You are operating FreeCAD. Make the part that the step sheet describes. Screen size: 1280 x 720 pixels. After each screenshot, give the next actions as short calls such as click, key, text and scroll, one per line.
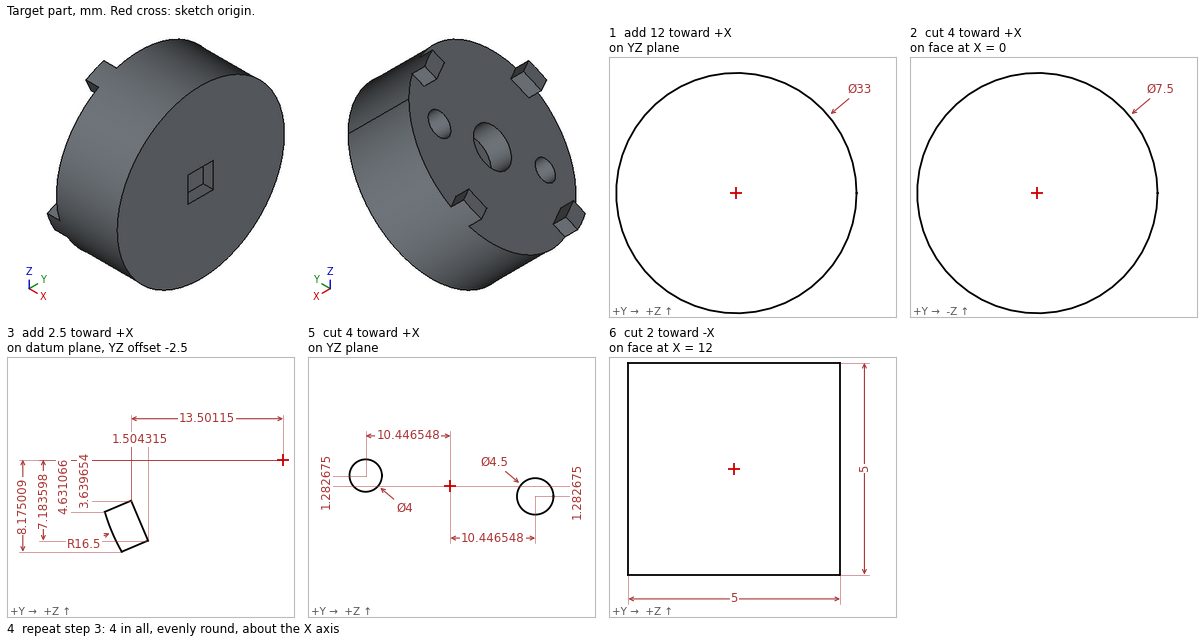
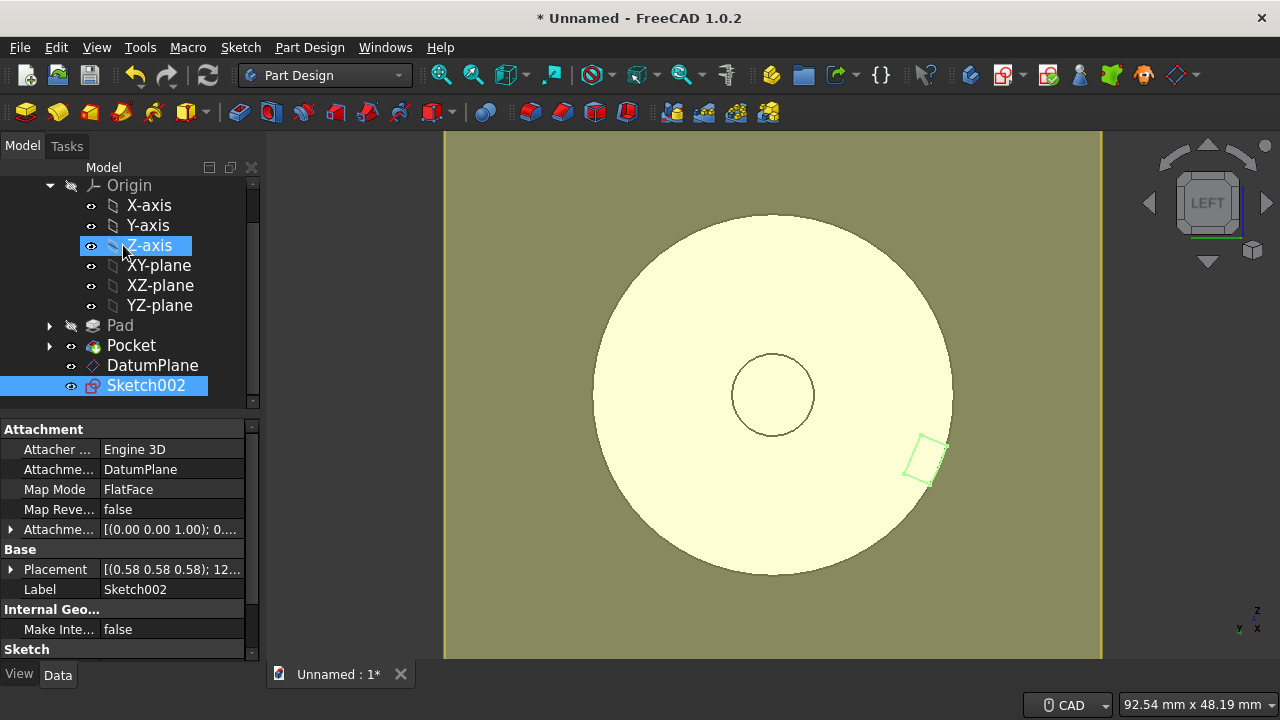
click(26, 112)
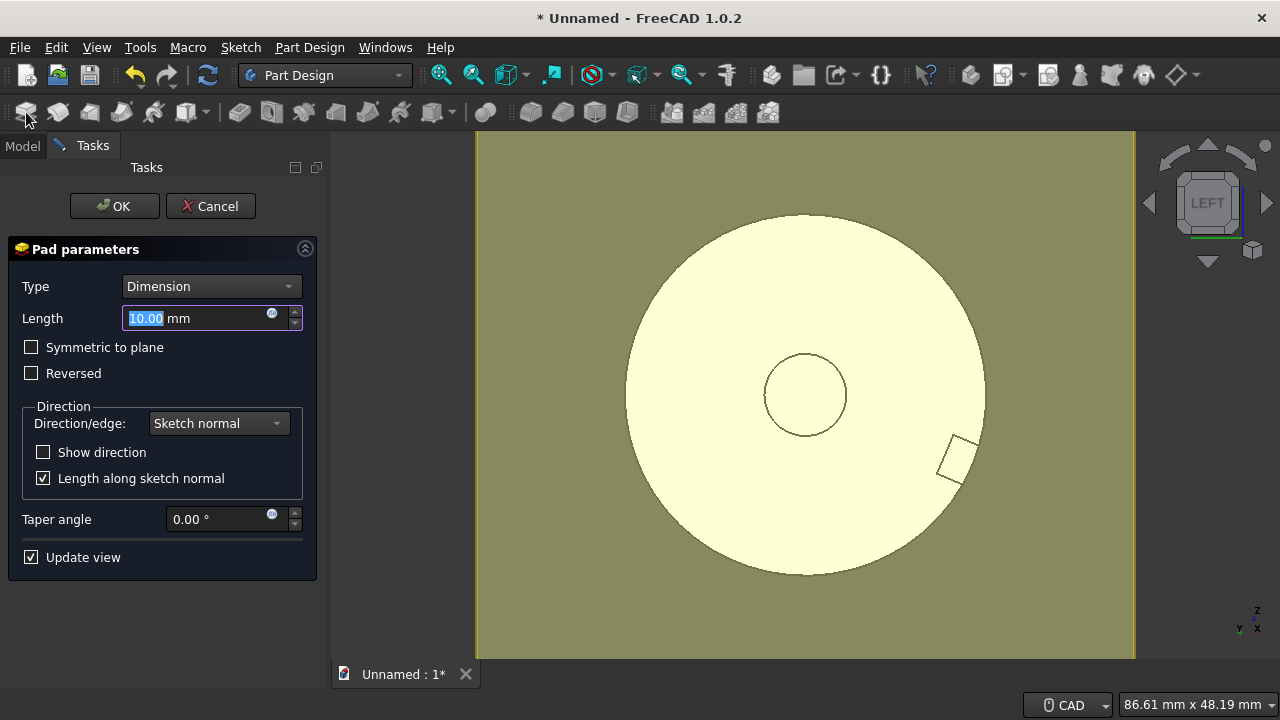
text(2.5)
key(Tab)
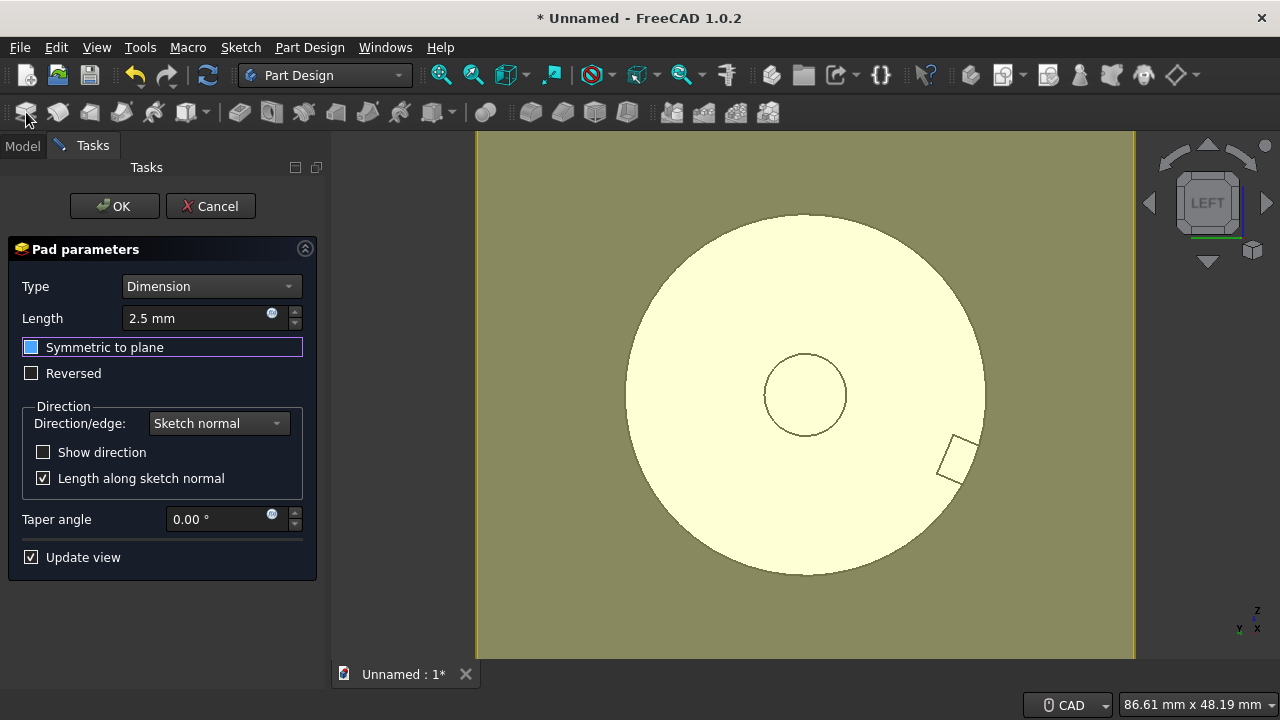
click(115, 206)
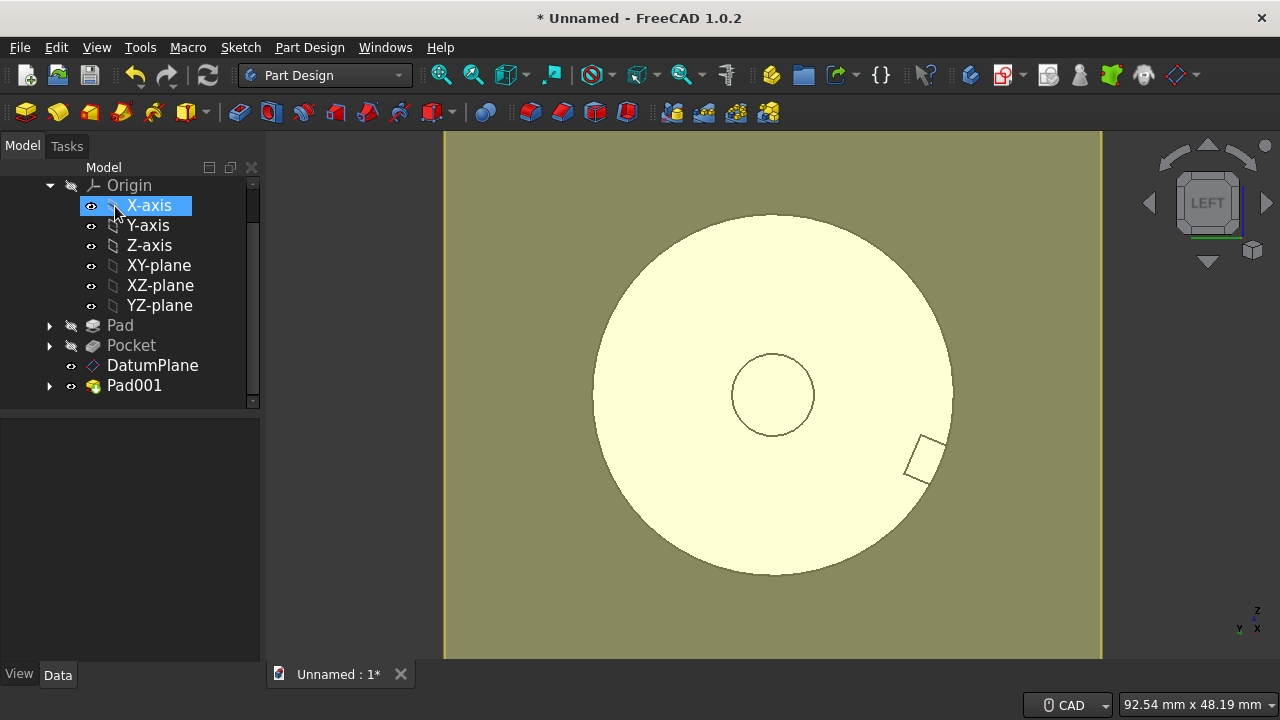
click(116, 366)
key(space)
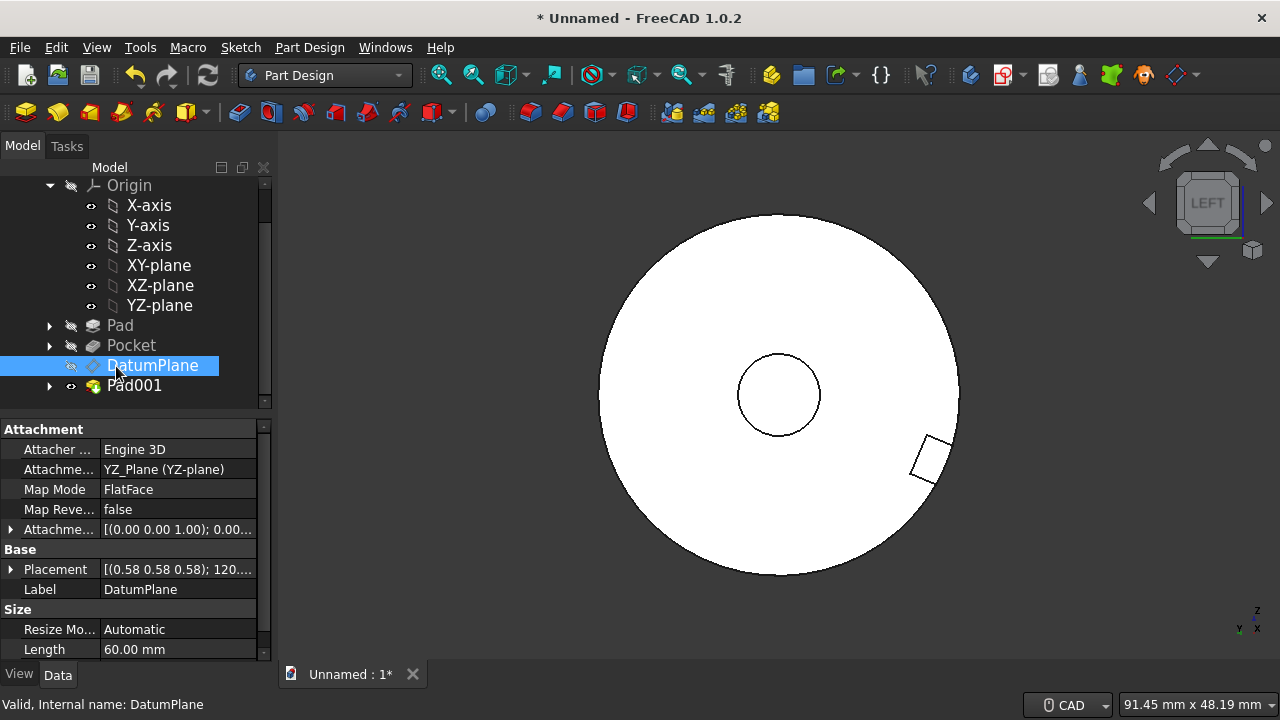
click(116, 386)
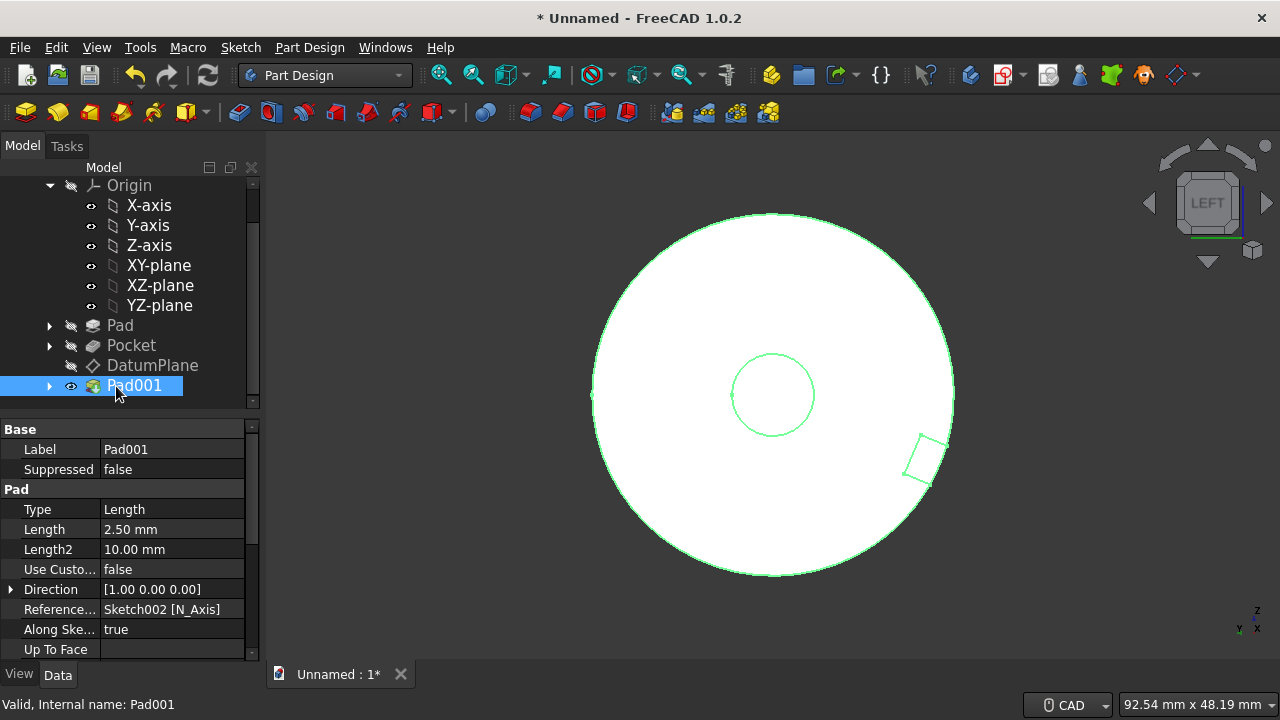
click(736, 112)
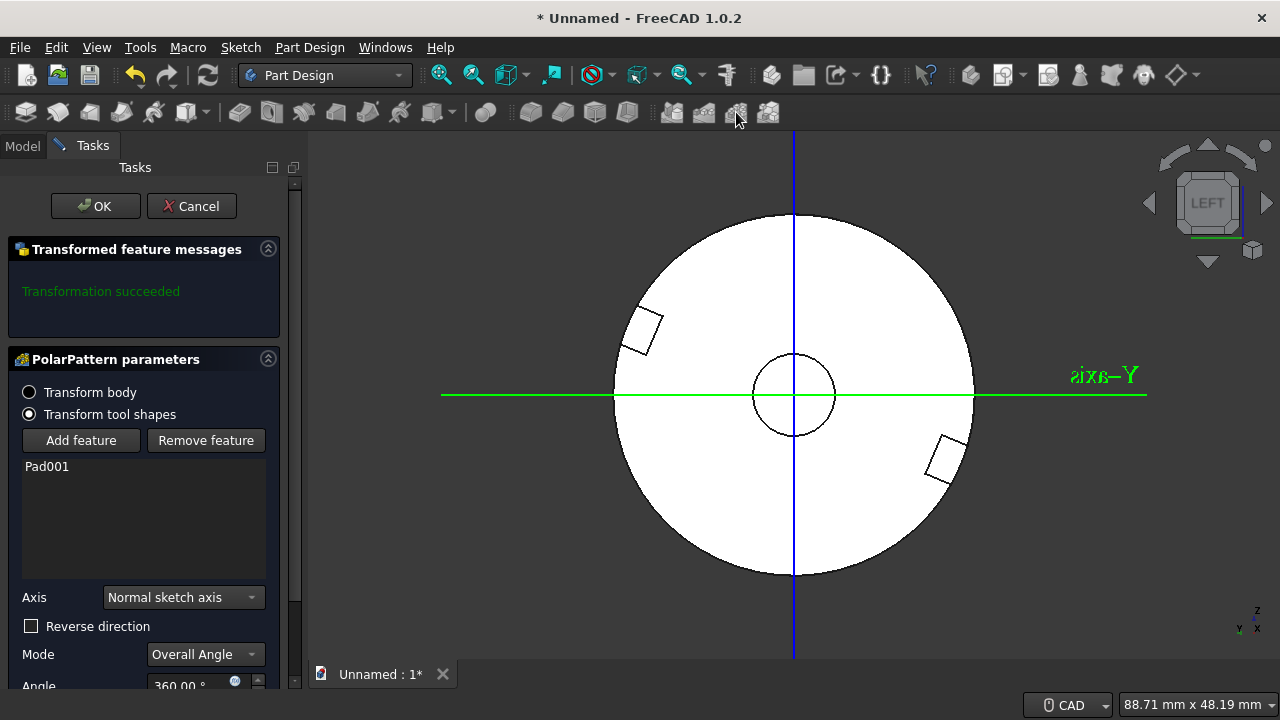
click(184, 598)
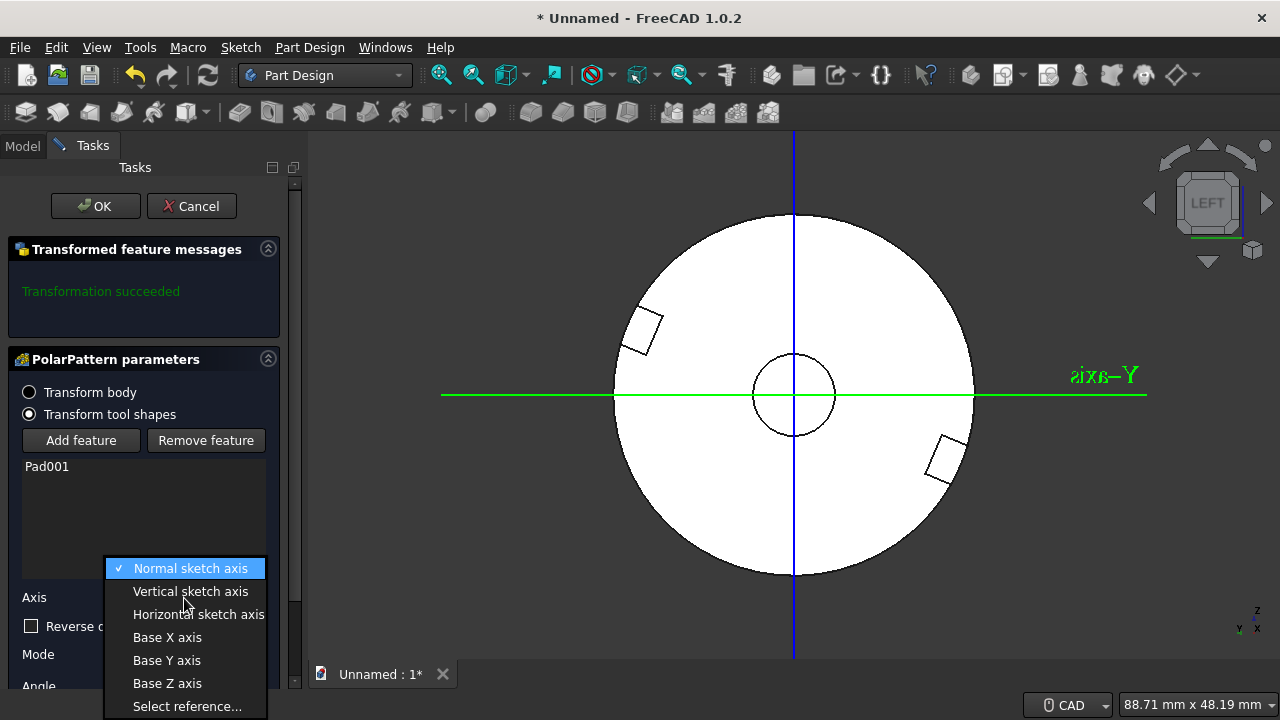
click(184, 638)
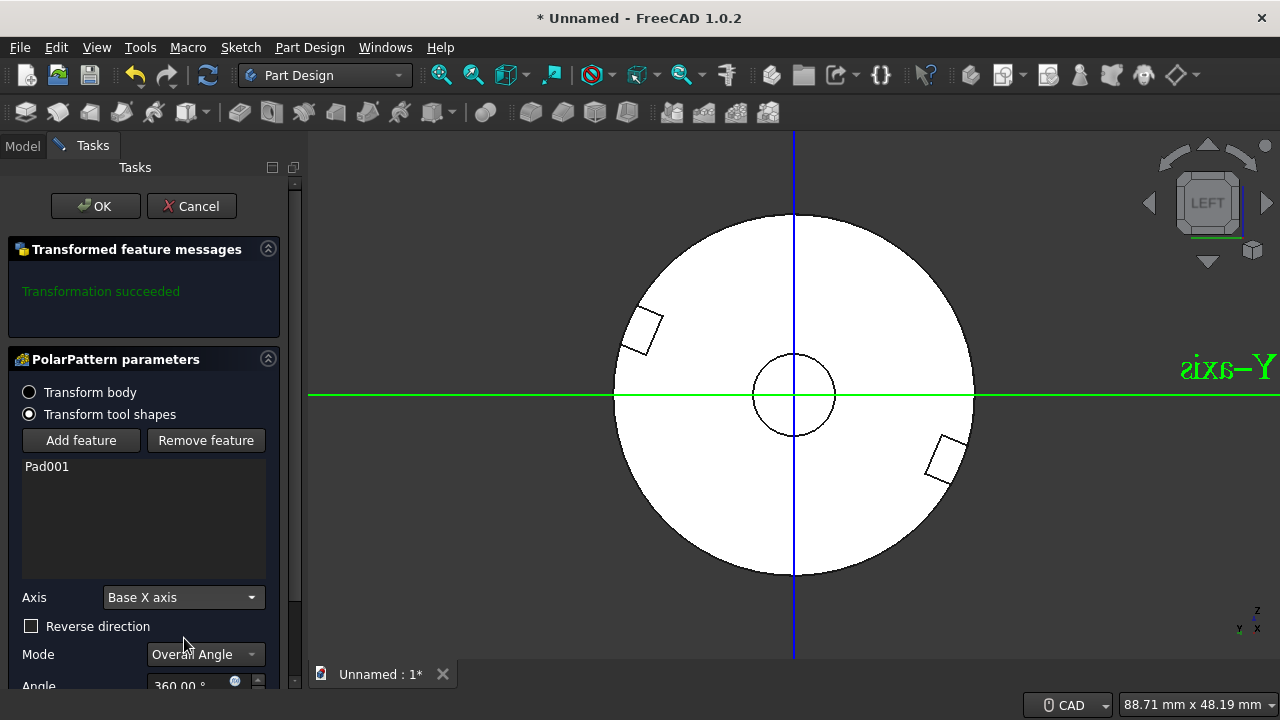
scroll(295, 432, down, 2)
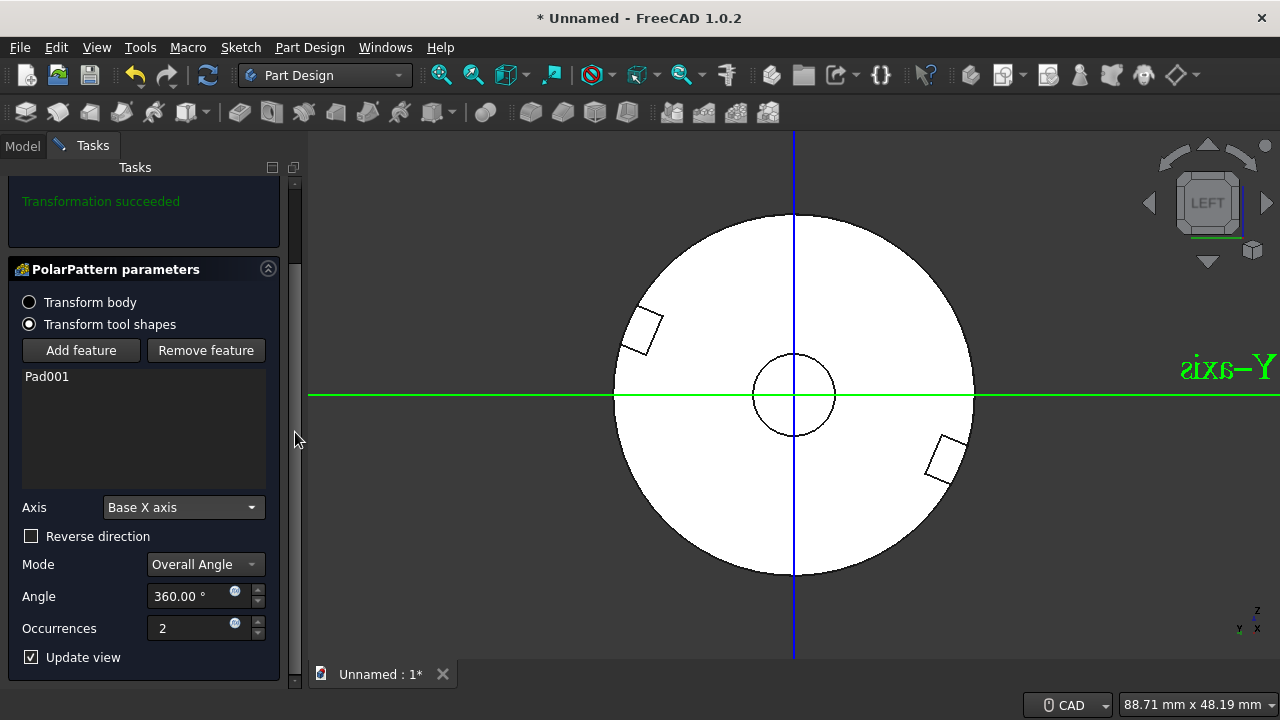
triple_click(198, 628)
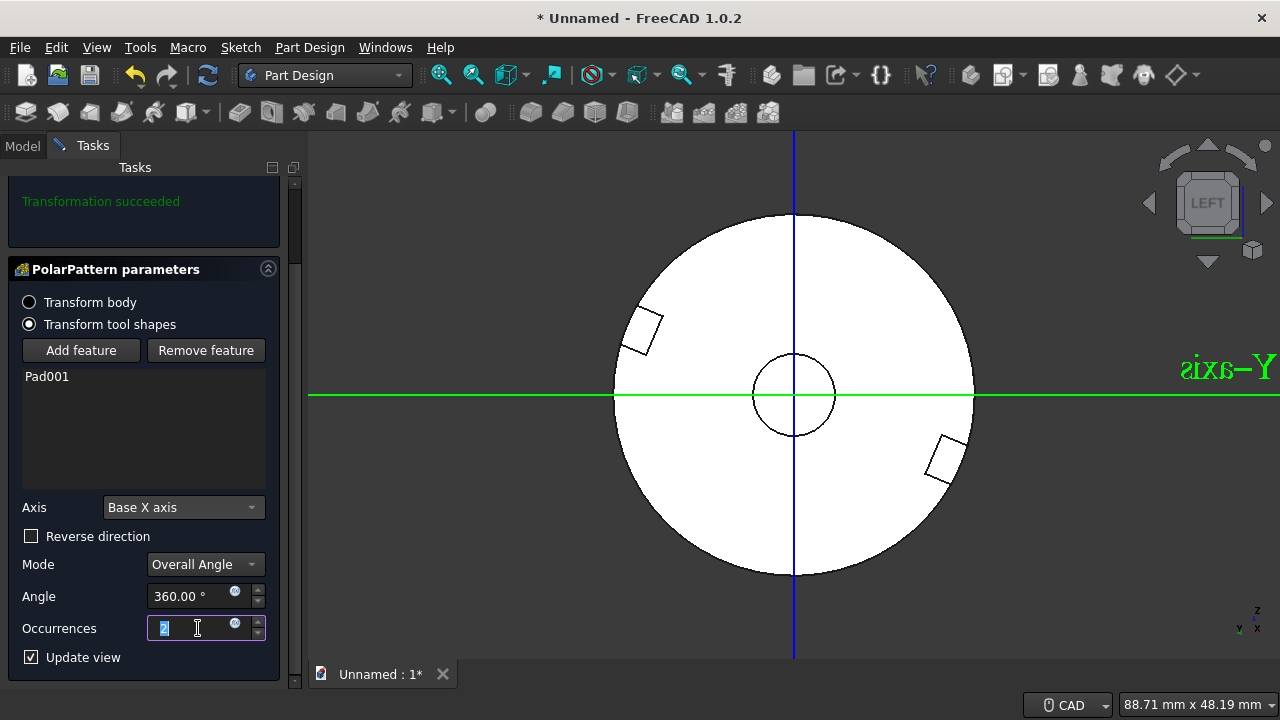
text(4)
key(Tab)